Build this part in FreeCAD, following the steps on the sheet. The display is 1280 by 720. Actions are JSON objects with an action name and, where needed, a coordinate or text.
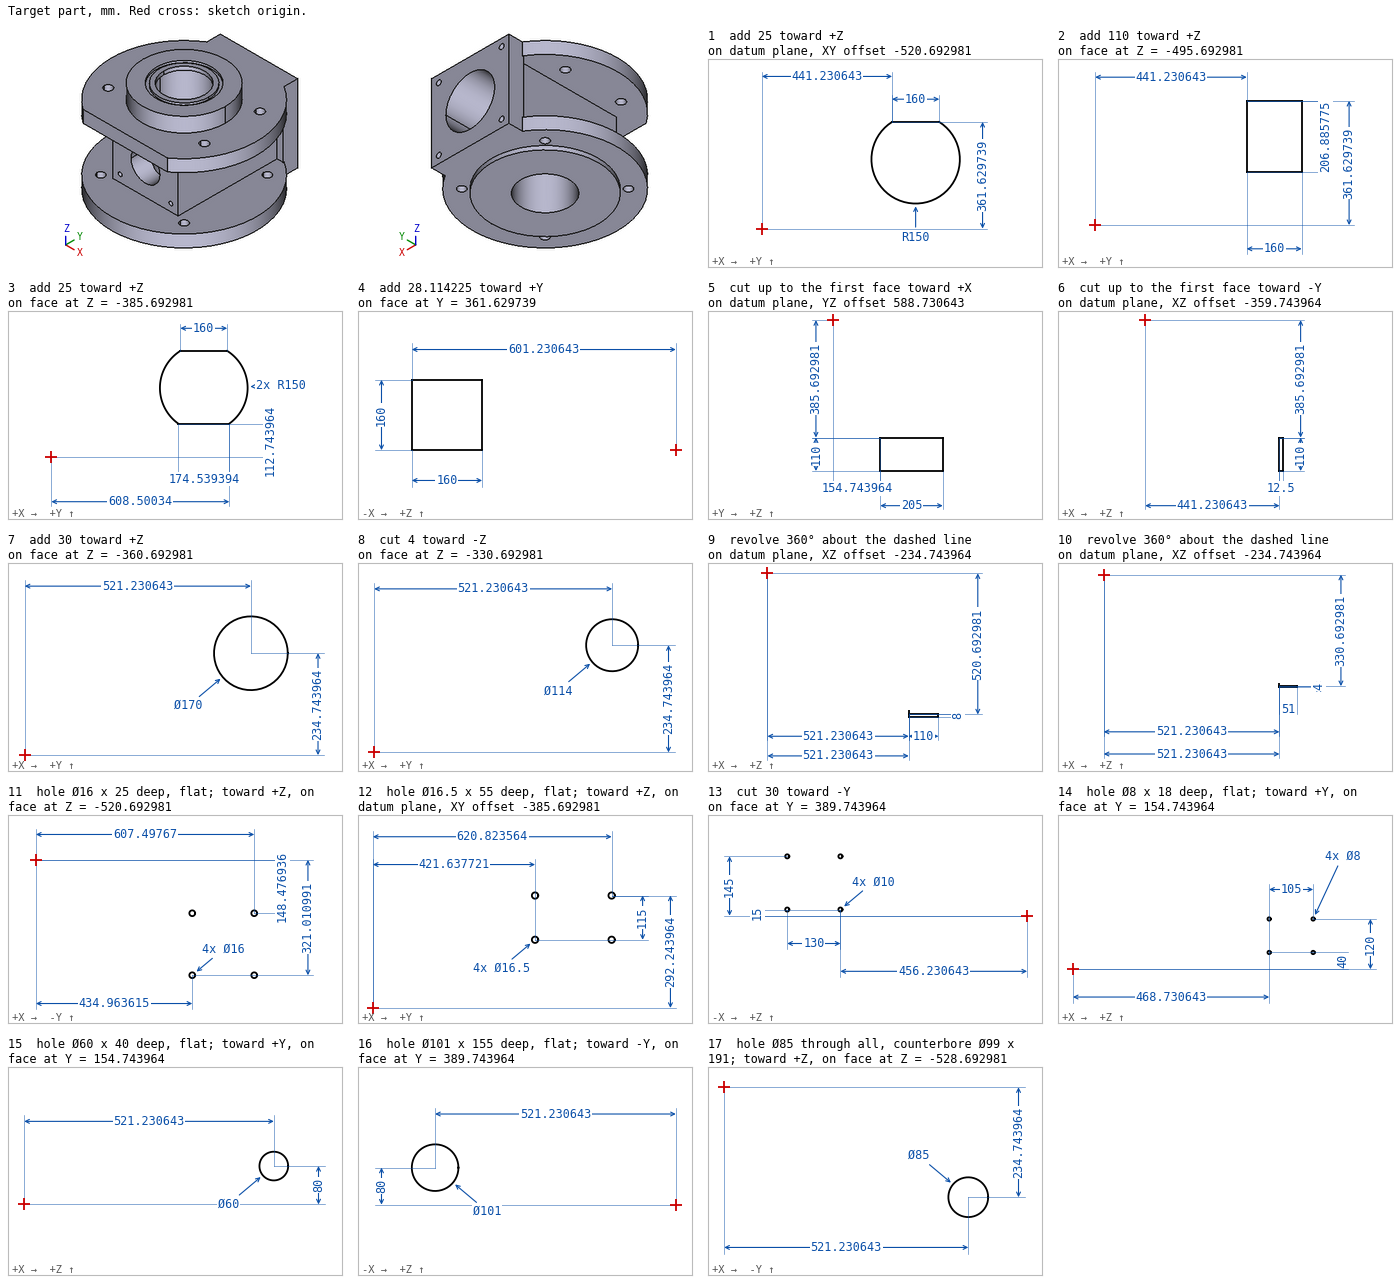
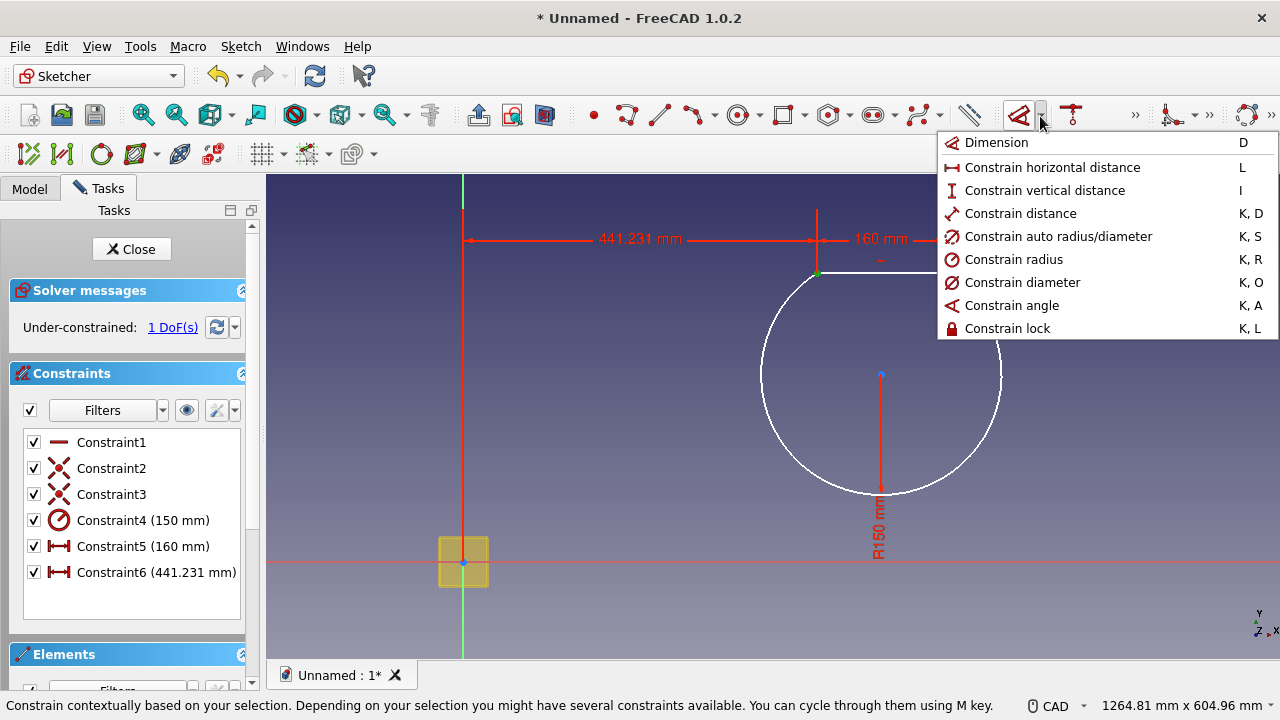
{"action": "left_click", "coordinate": [1108, 190]}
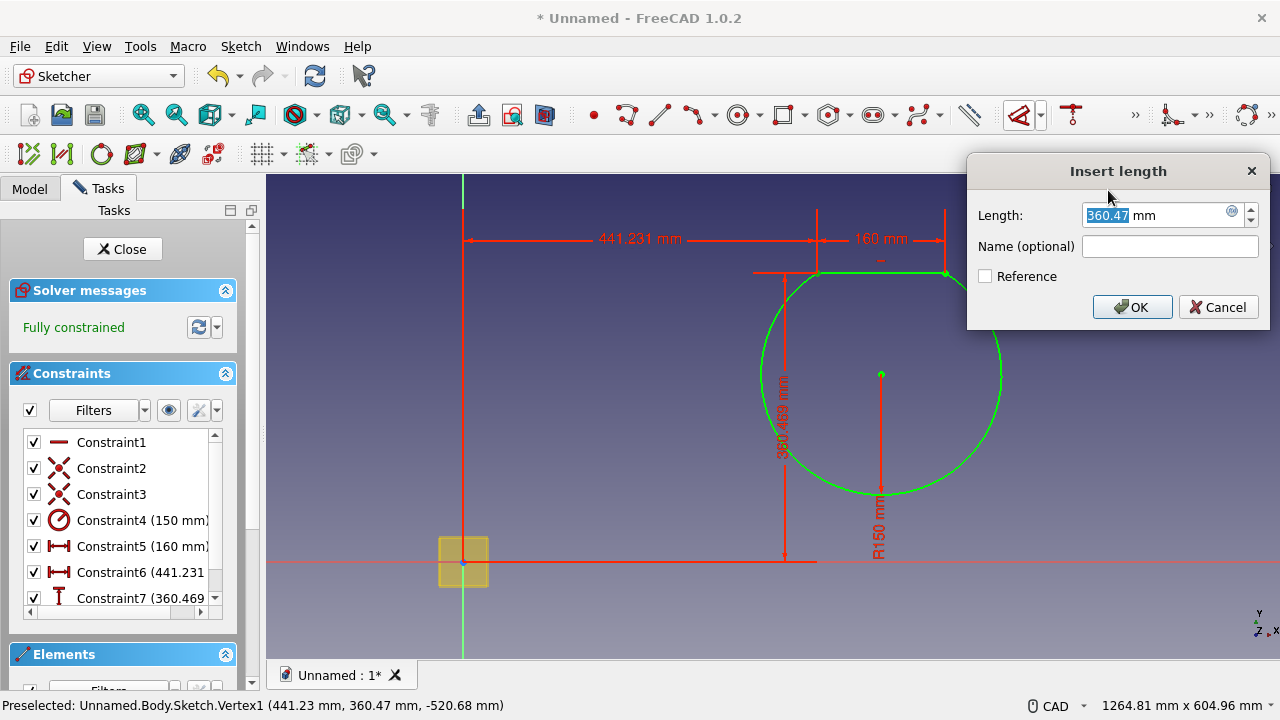
{"action": "type", "text": "361.629739"}
{"action": "key", "text": "Return"}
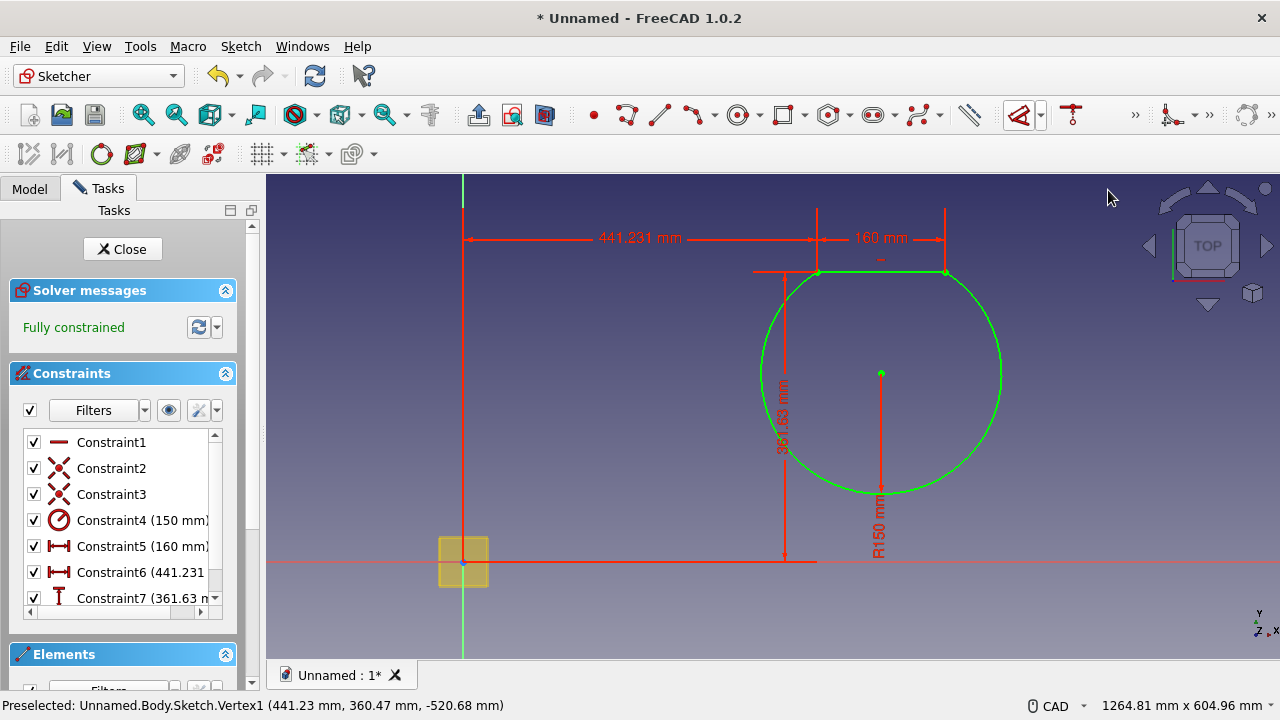
{"action": "left_click", "coordinate": [123, 249]}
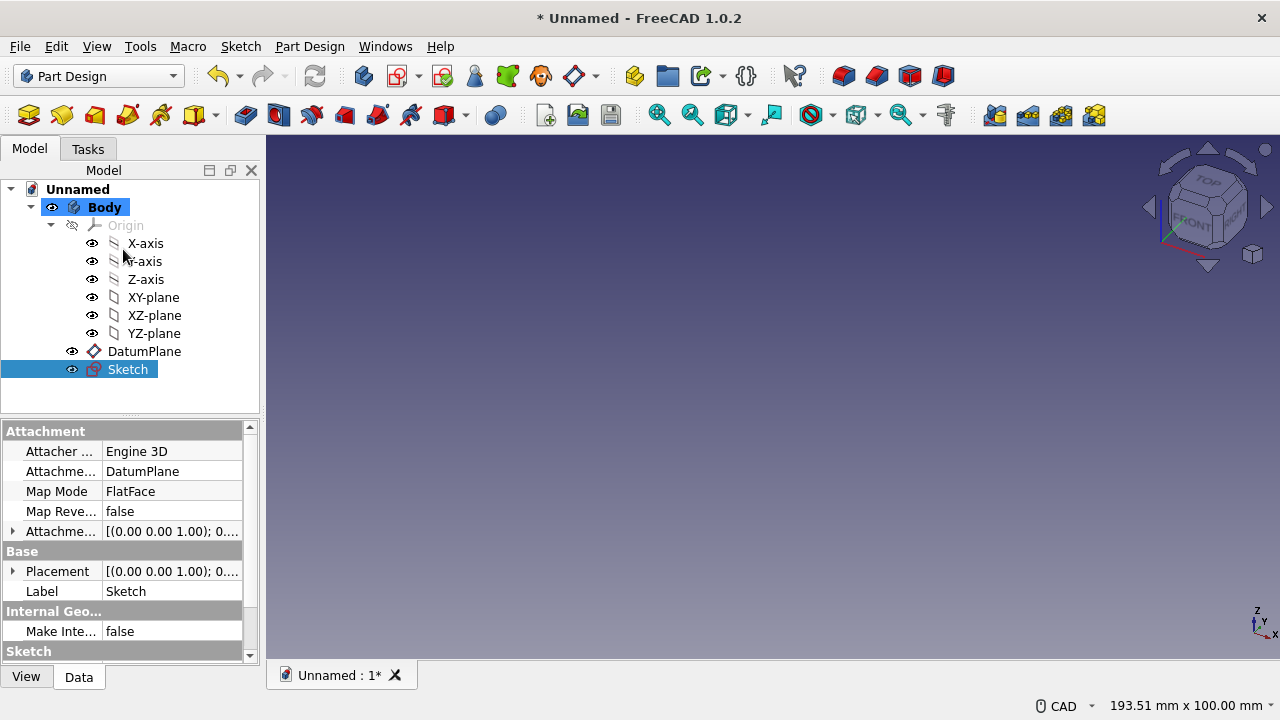
{"action": "left_click", "coordinate": [29, 116]}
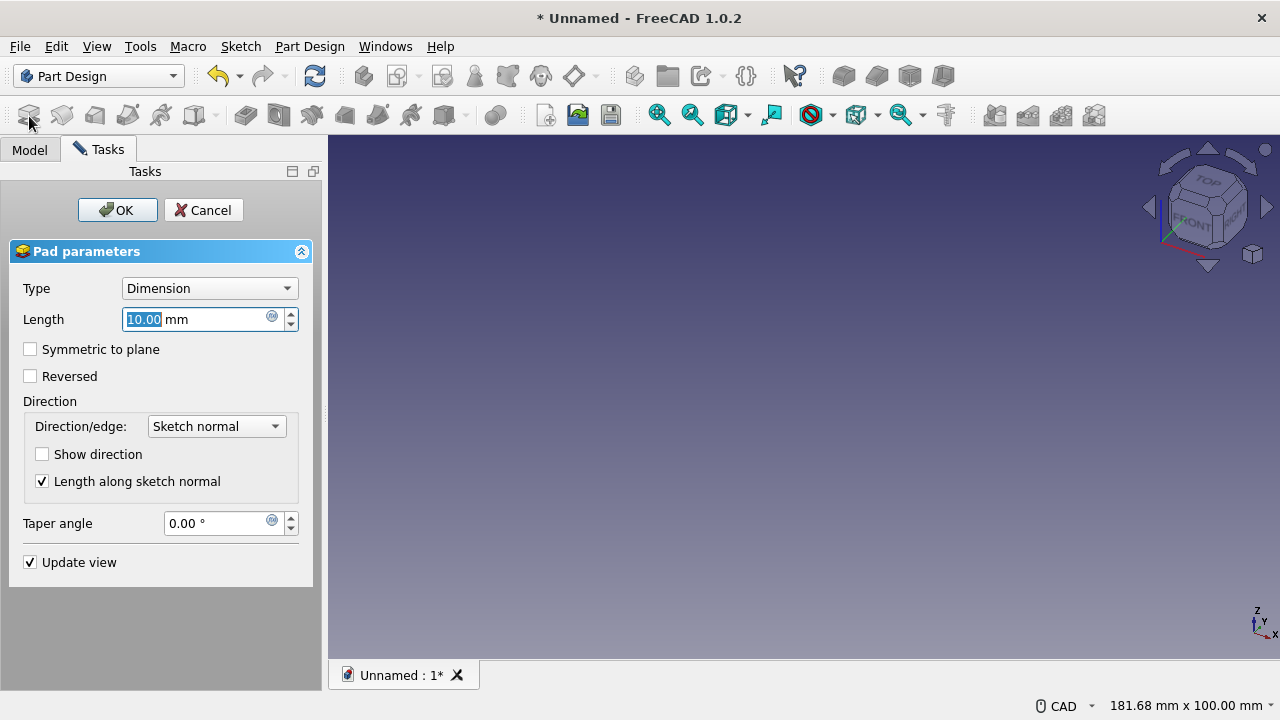
{"action": "type", "text": "25"}
{"action": "key", "text": "Tab"}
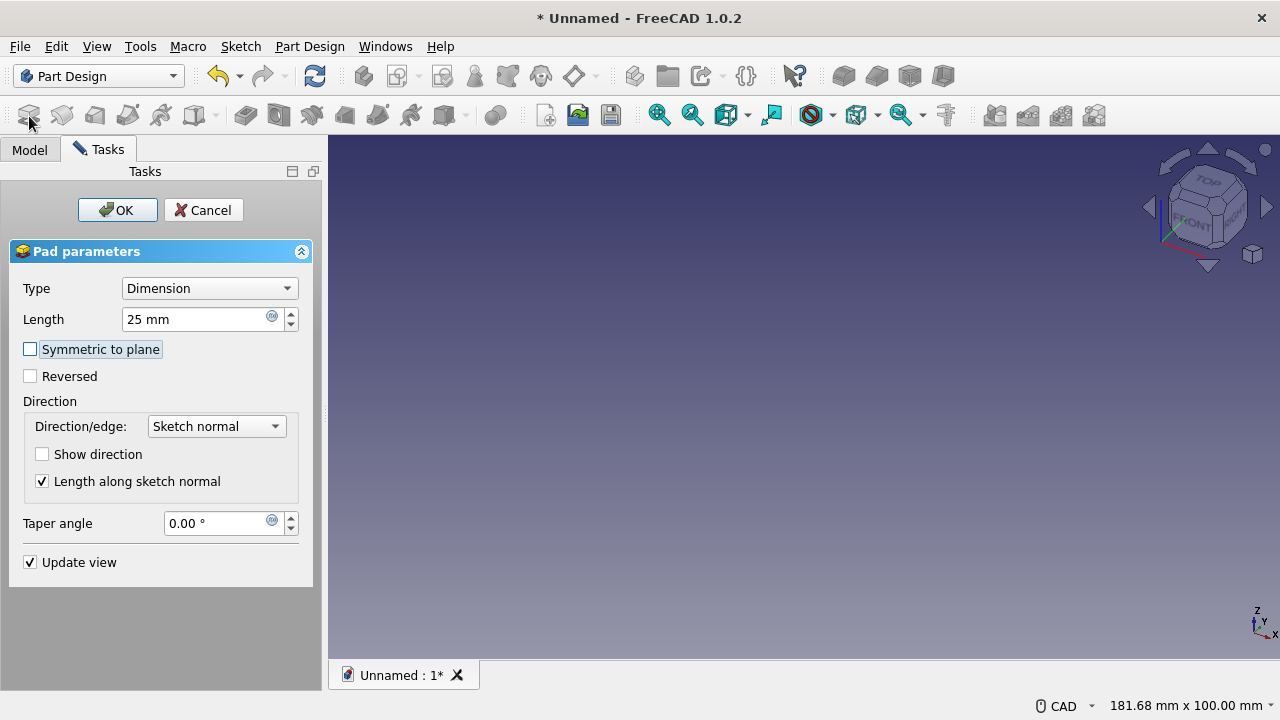
{"action": "left_click", "coordinate": [118, 210]}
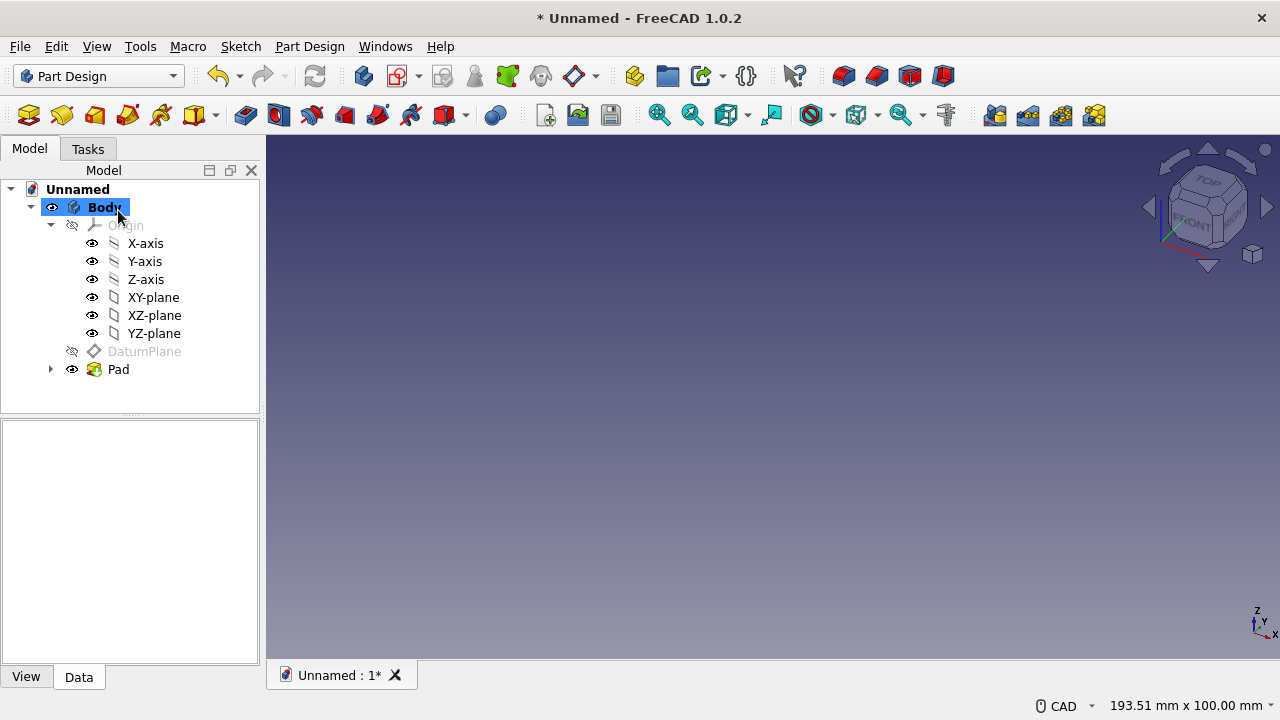
{"action": "left_click", "coordinate": [660, 116]}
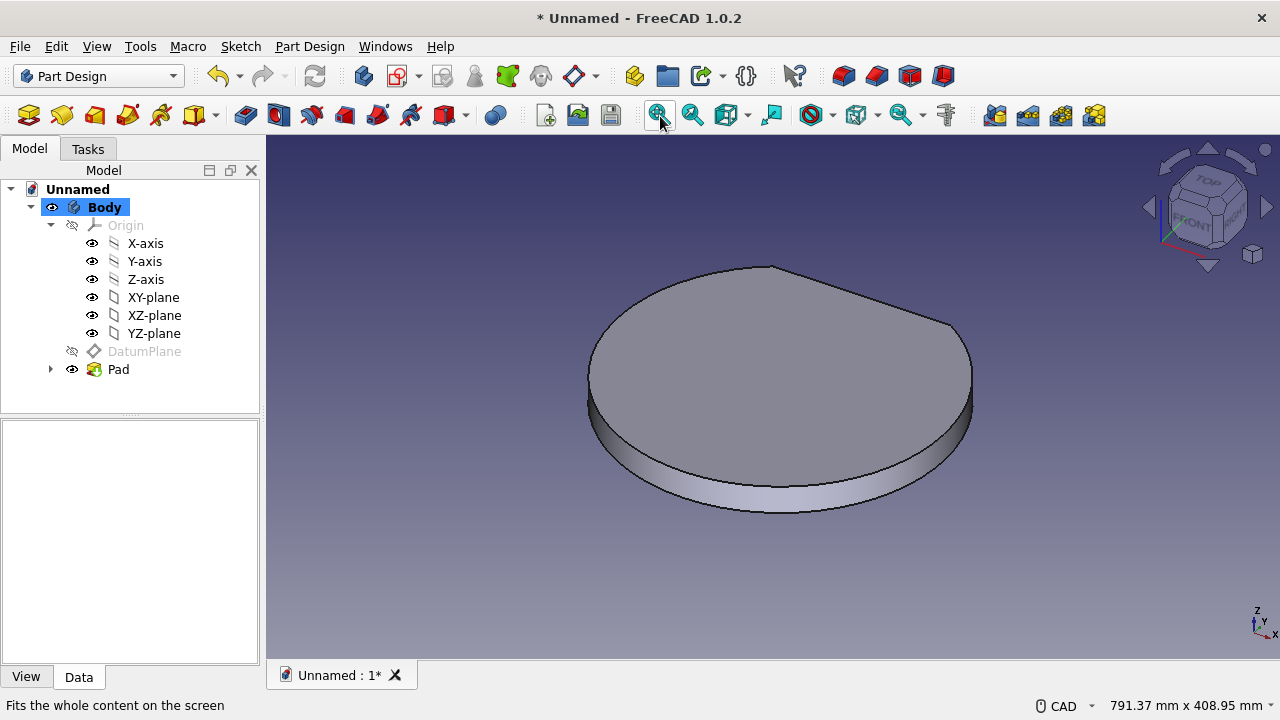
{"action": "left_click", "coordinate": [773, 383]}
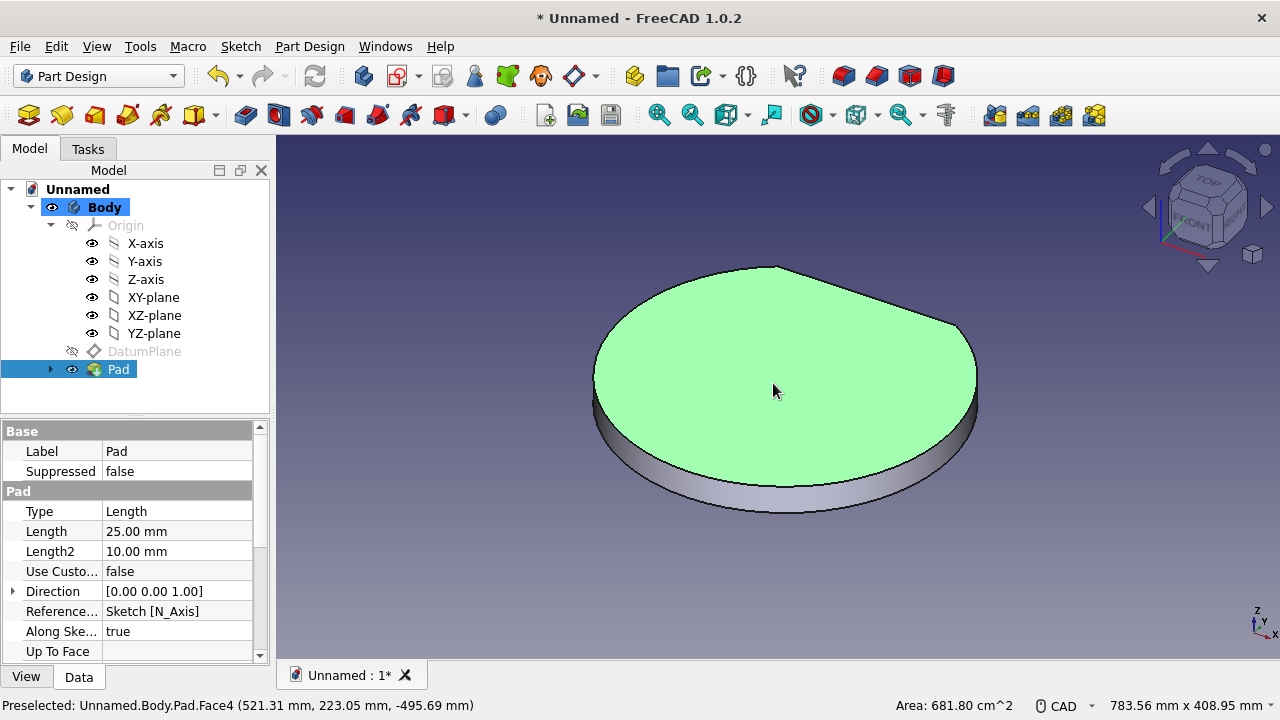
{"action": "left_click", "coordinate": [396, 76]}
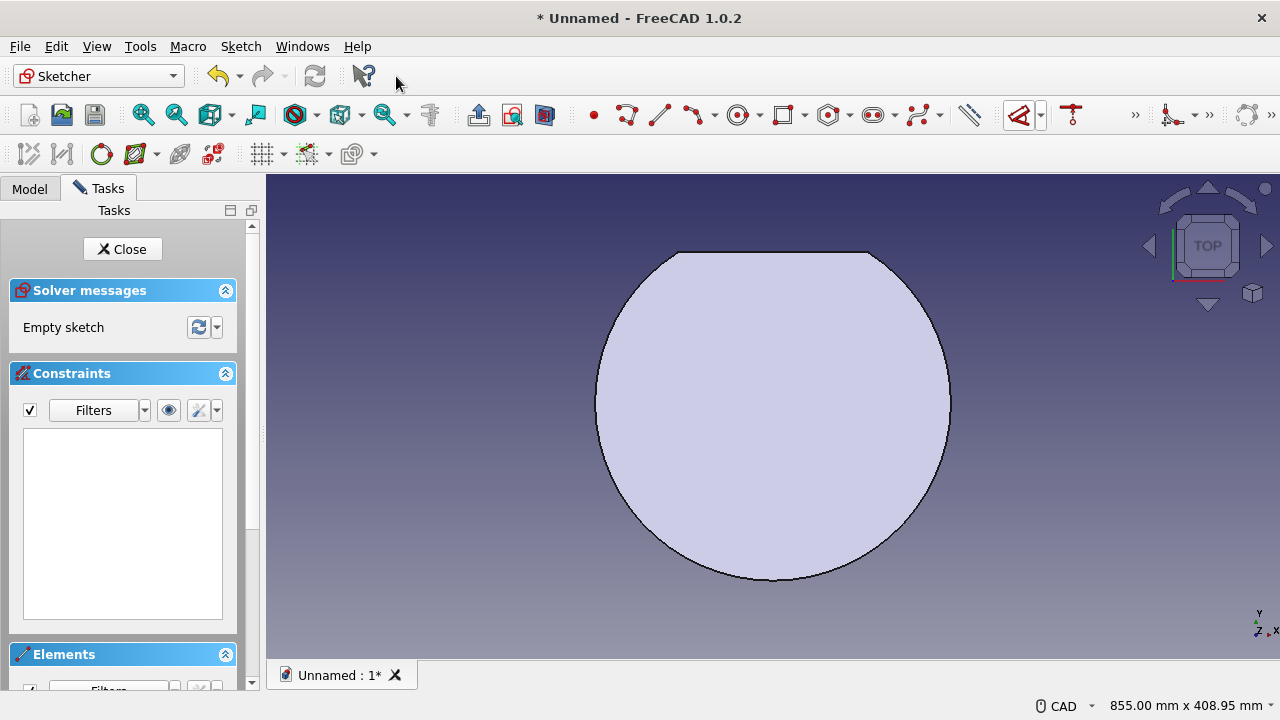
{"action": "left_click", "coordinate": [782, 116]}